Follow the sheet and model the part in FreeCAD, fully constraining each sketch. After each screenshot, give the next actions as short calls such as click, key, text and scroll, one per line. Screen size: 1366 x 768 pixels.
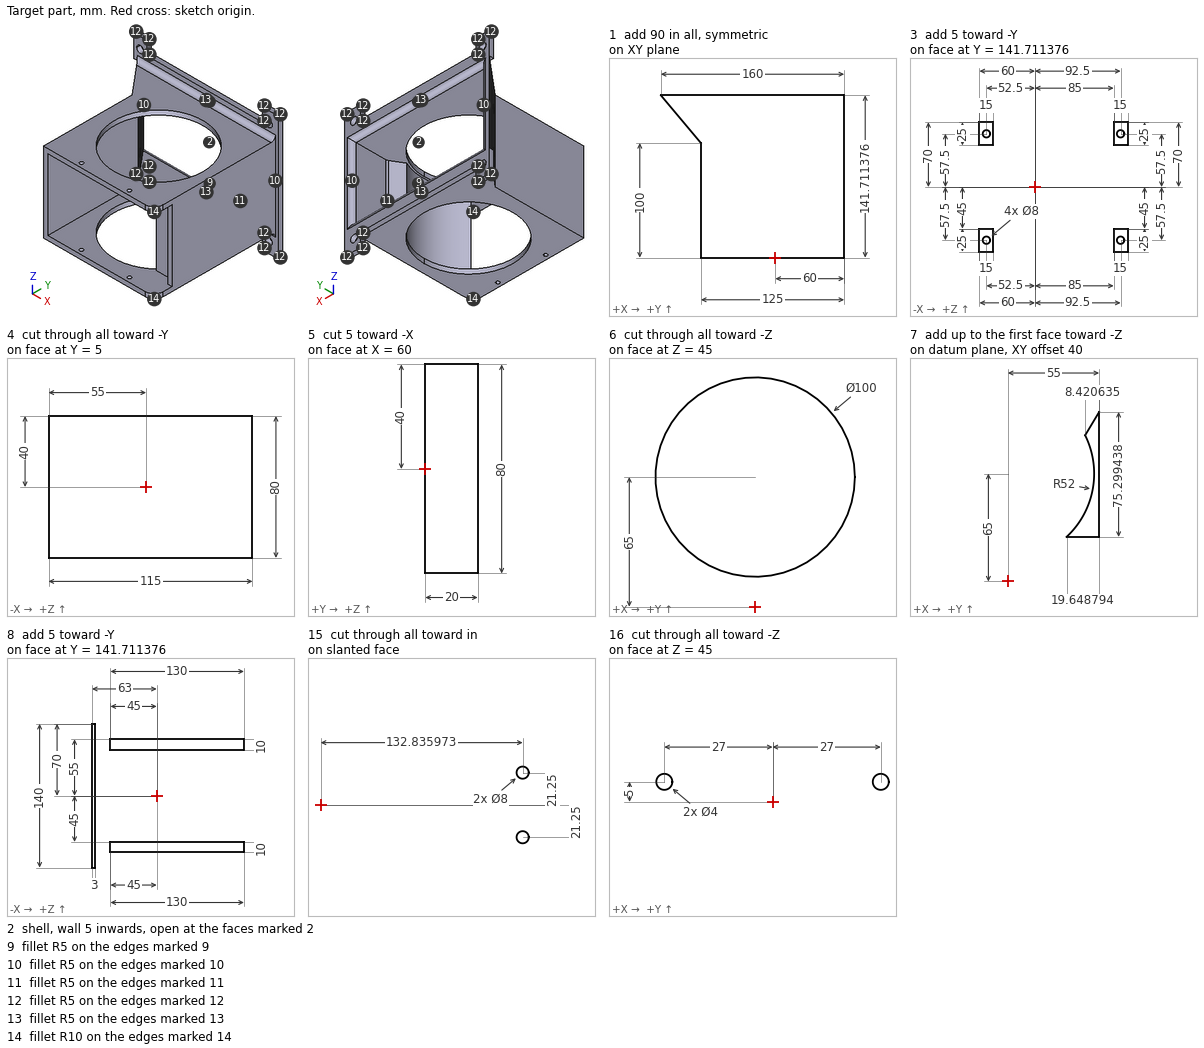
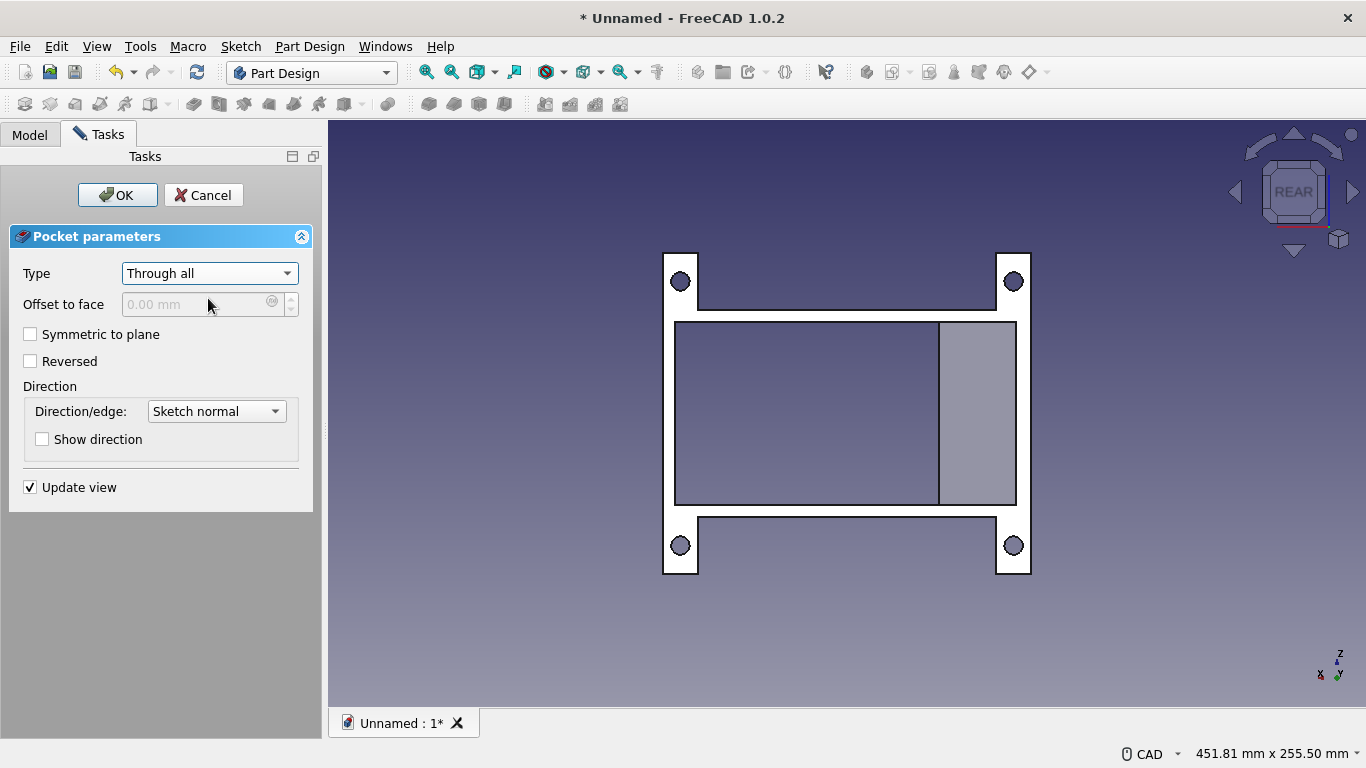
click(118, 195)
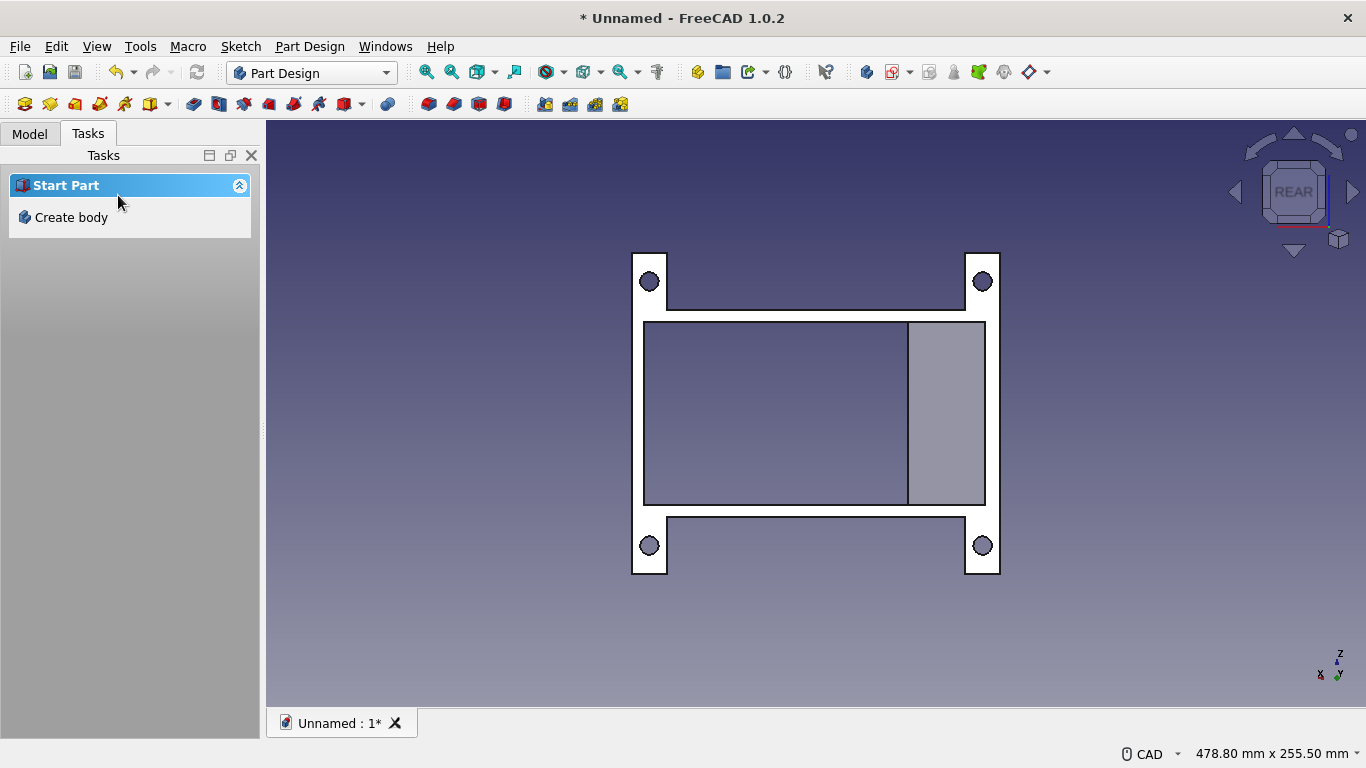
key(0)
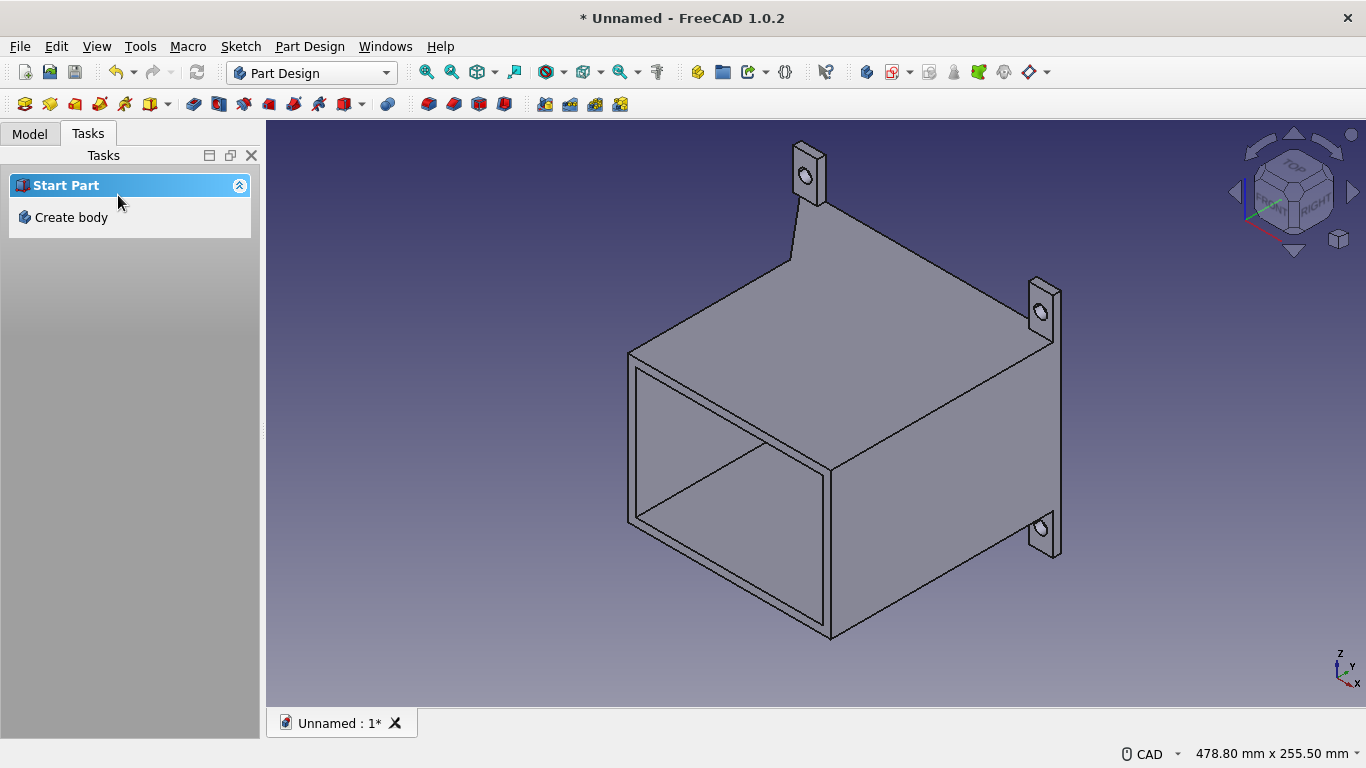
click(979, 469)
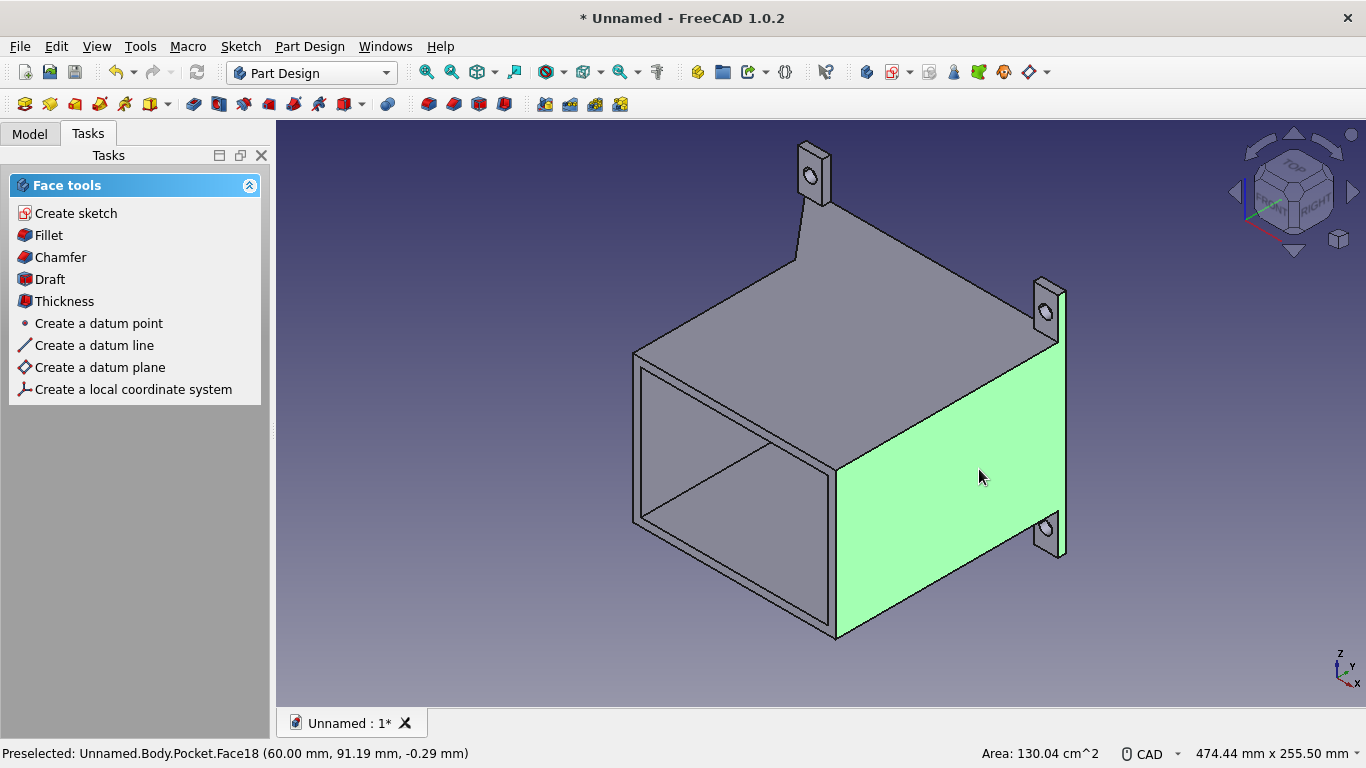
click(892, 72)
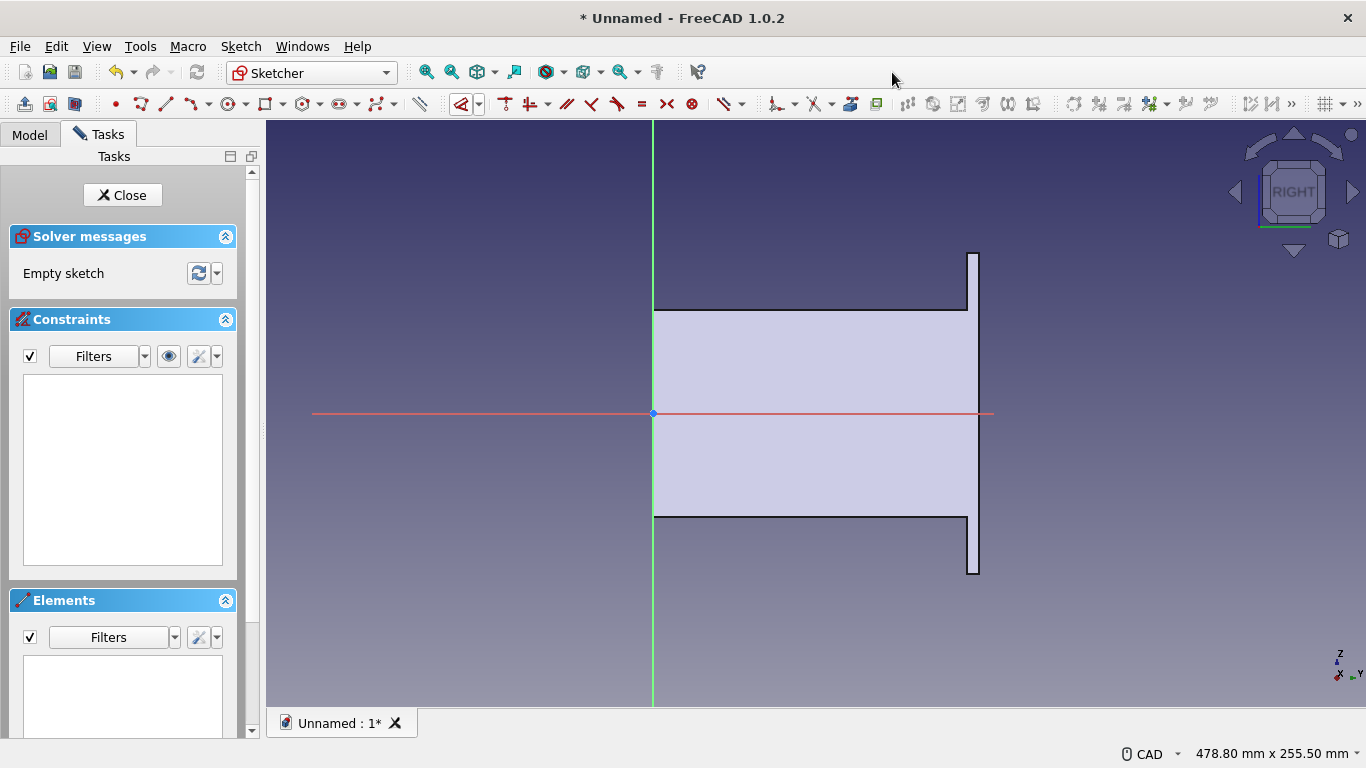
scroll(618, 413, up, 4)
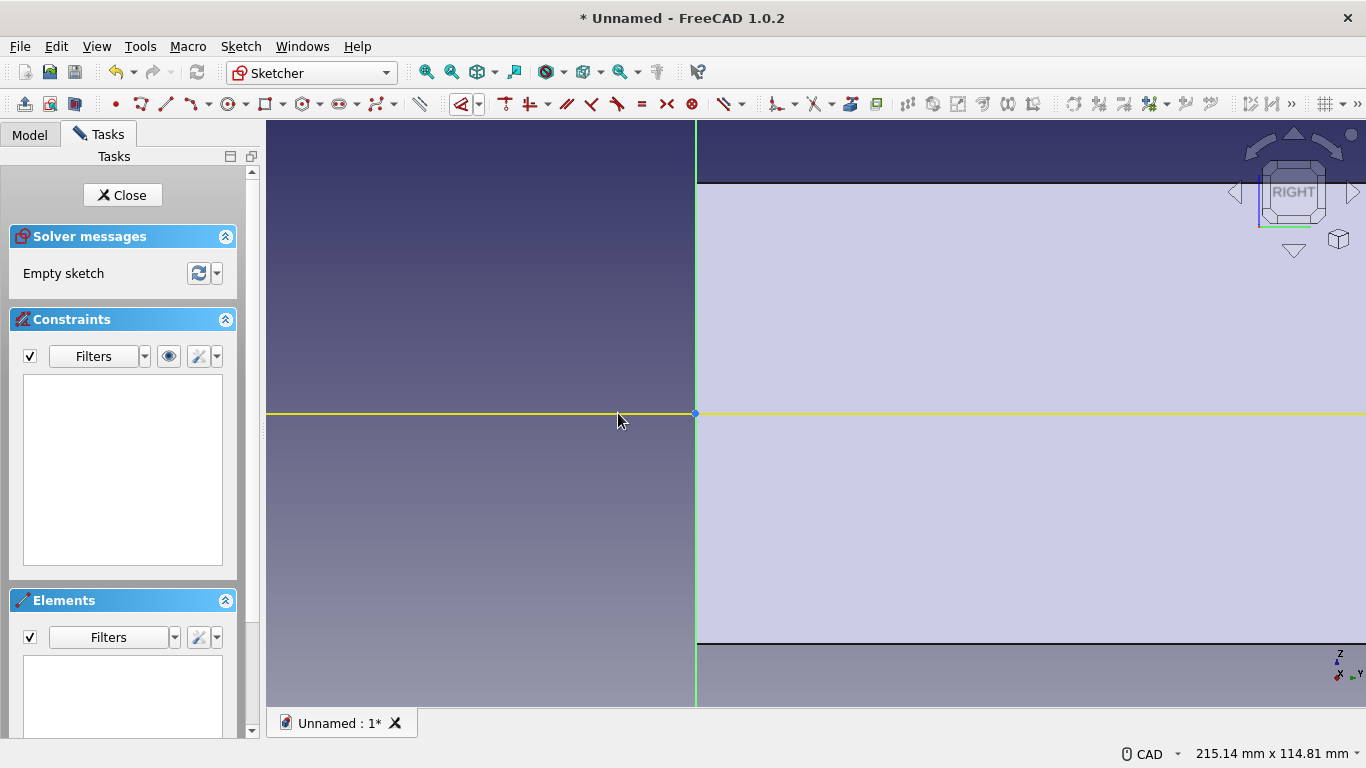
key(g)
key(r)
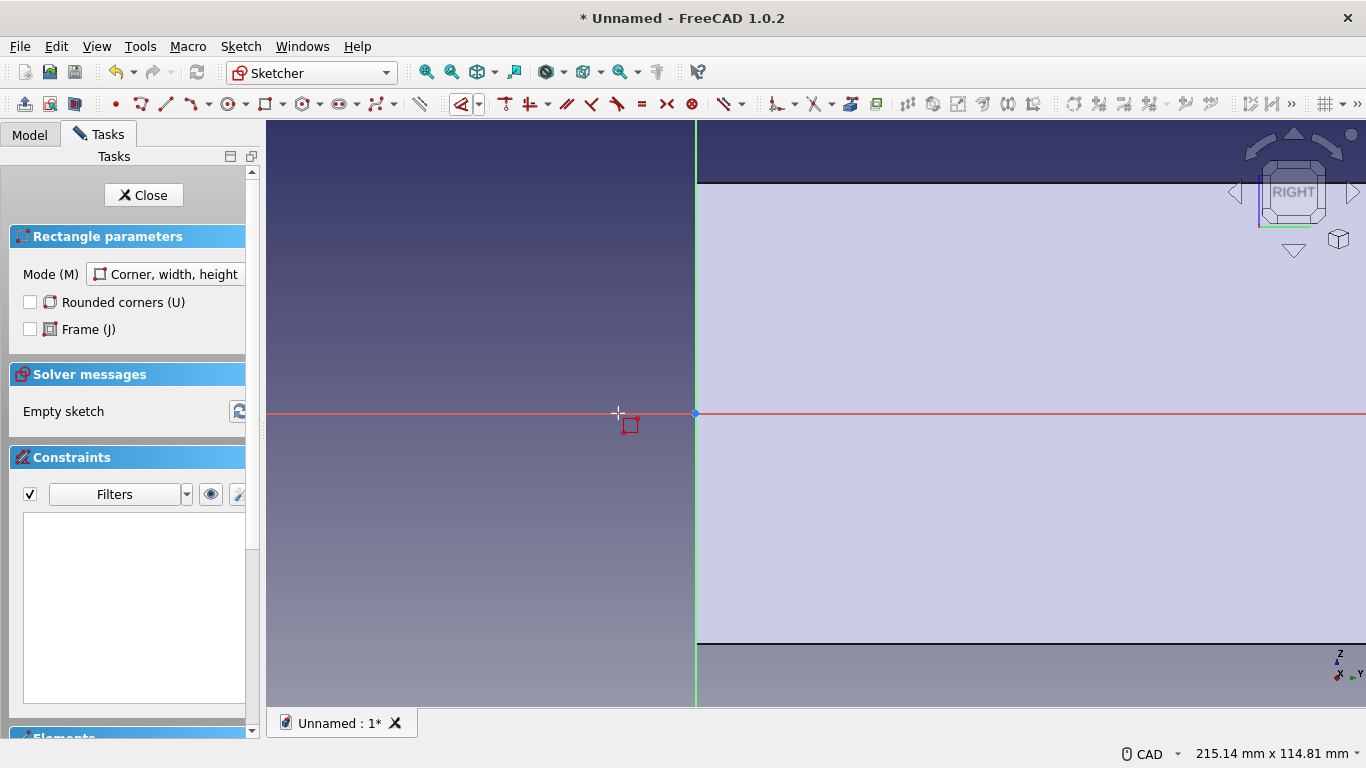
click(696, 209)
move(798, 618)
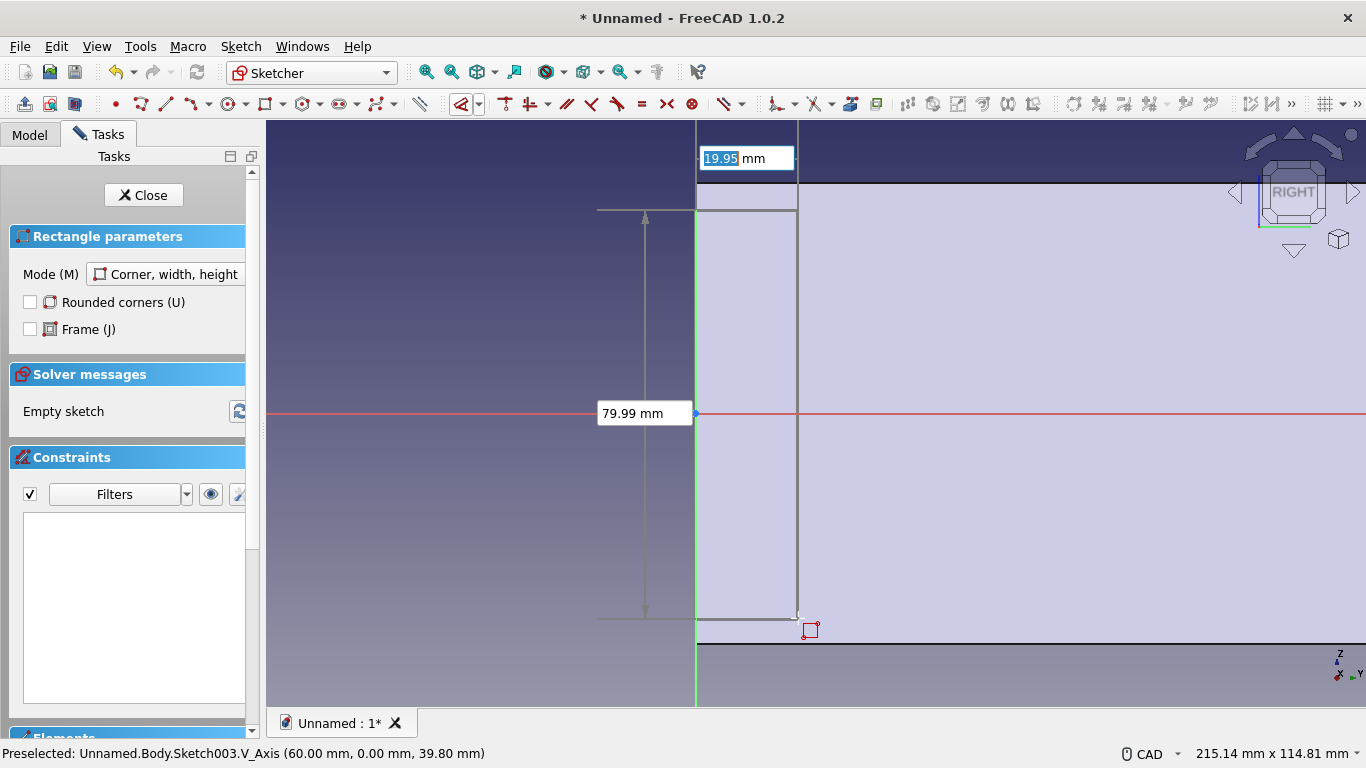
text(20)
key(Tab)
text(80)
key(Return)
key(Escape)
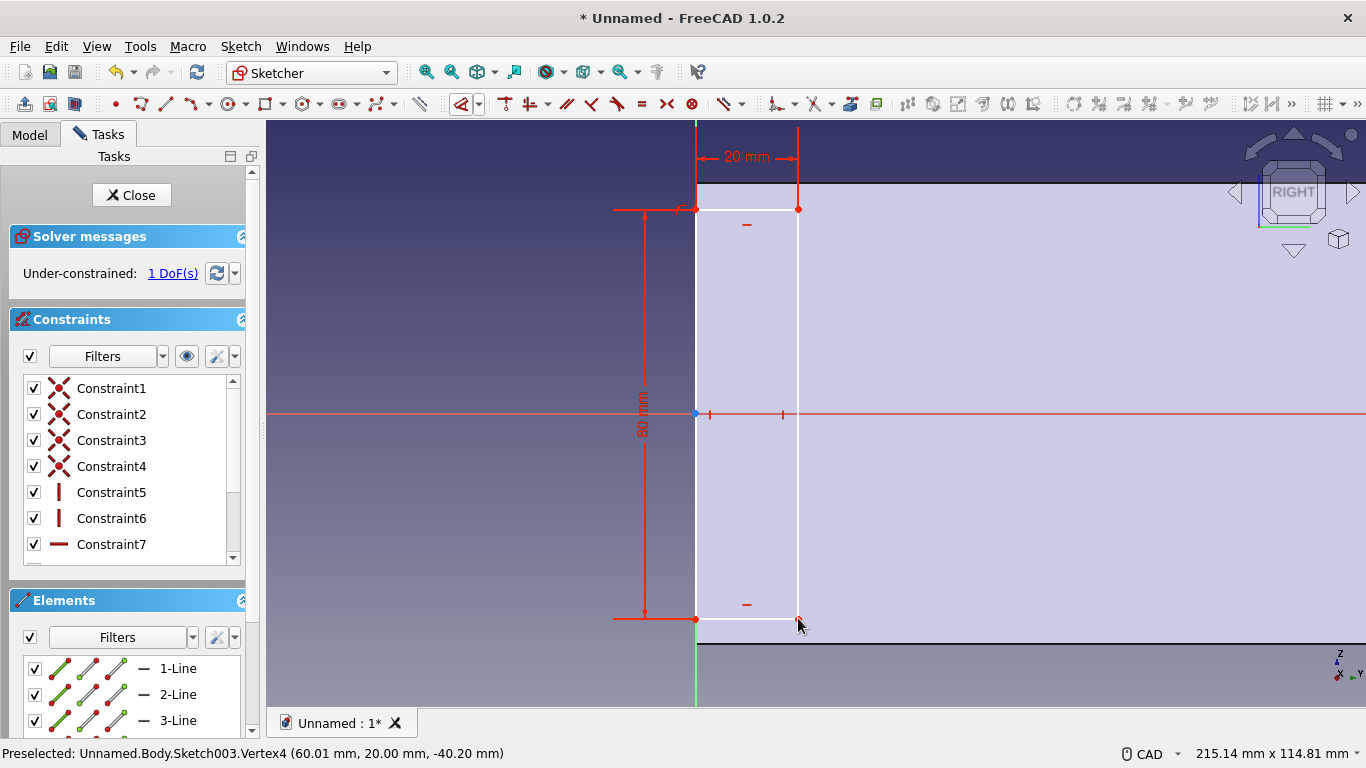
click(696, 210)